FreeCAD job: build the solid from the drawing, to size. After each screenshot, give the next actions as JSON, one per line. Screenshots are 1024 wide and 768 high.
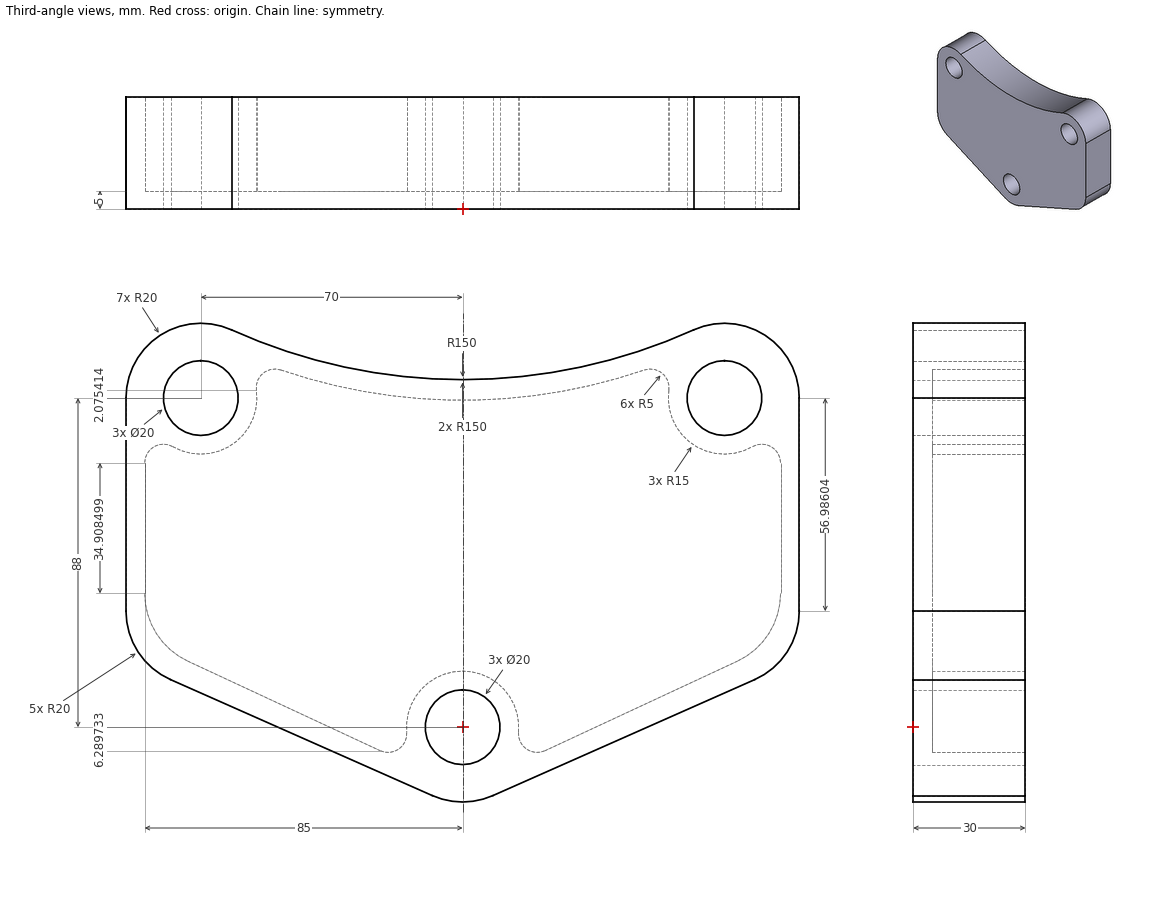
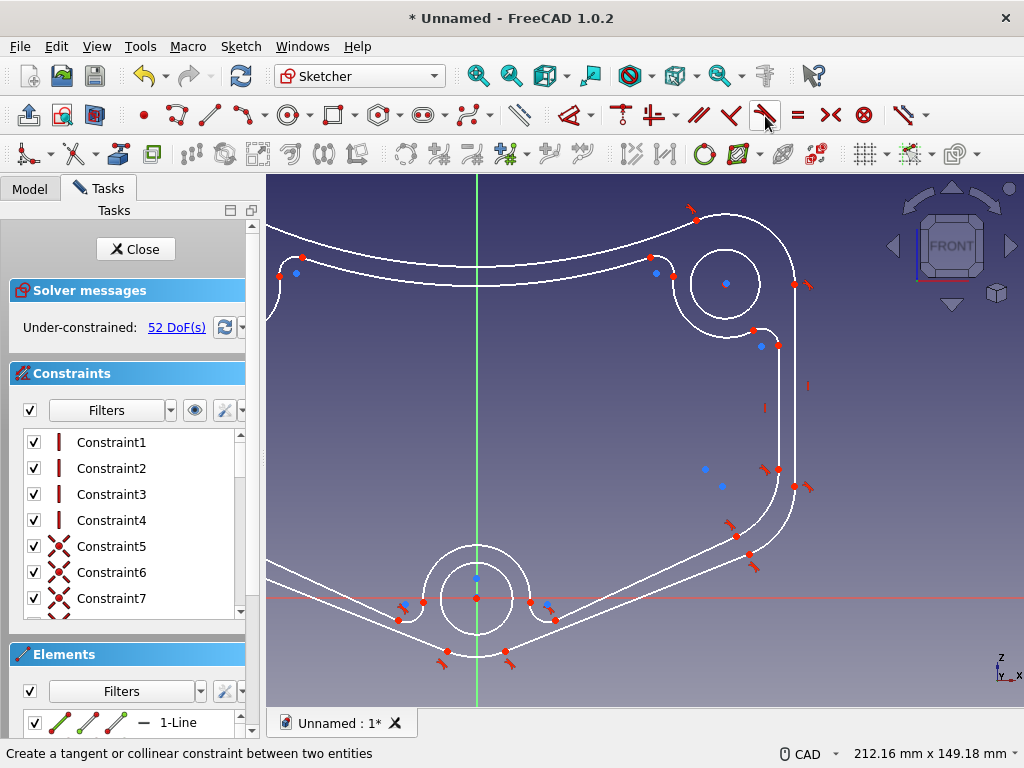
{"action": "left_click", "coordinate": [779, 433]}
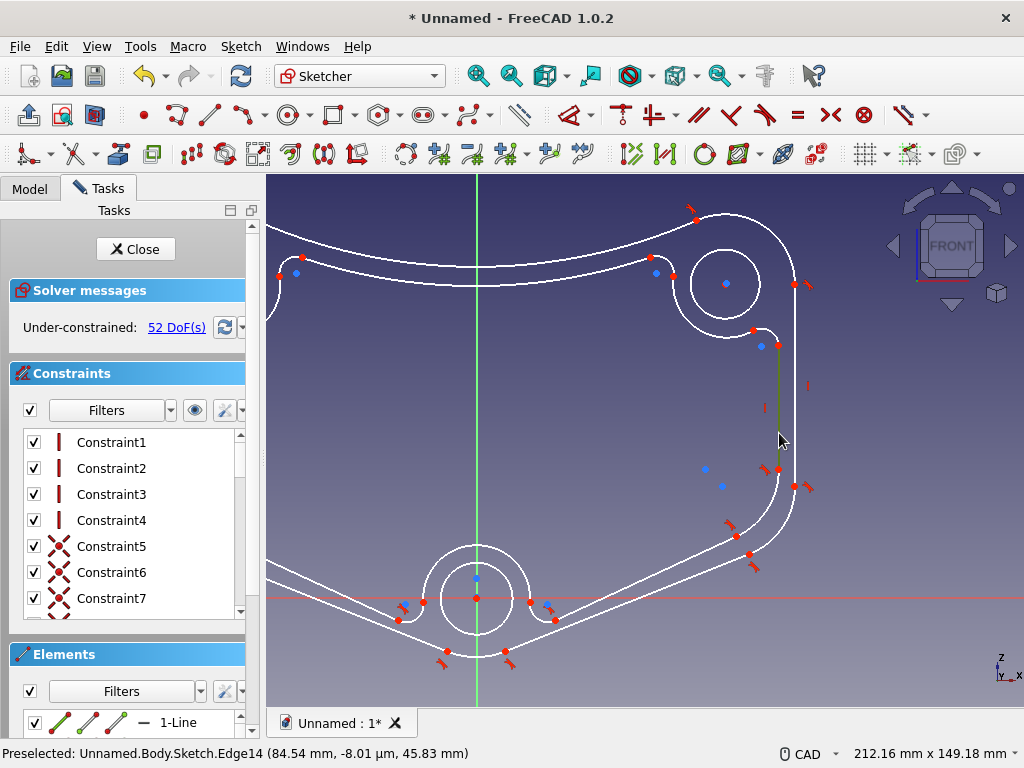
{"action": "scroll", "coordinate": [776, 336], "scroll_direction": "up", "scroll_amount": 2}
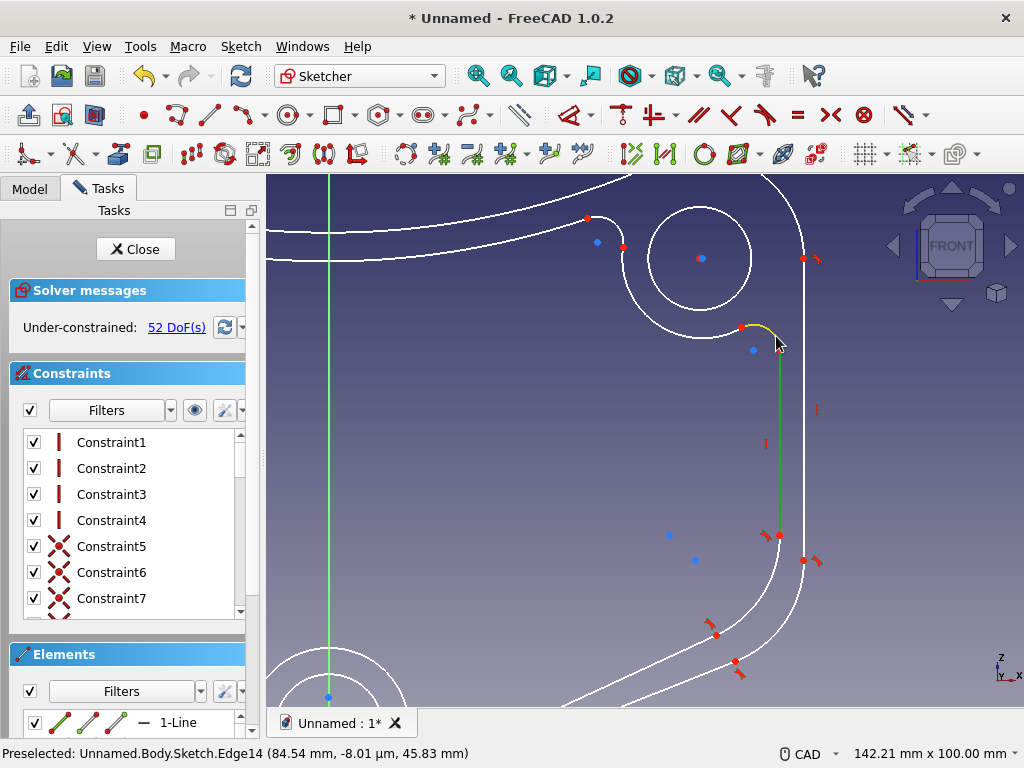
{"action": "left_click", "coordinate": [775, 336]}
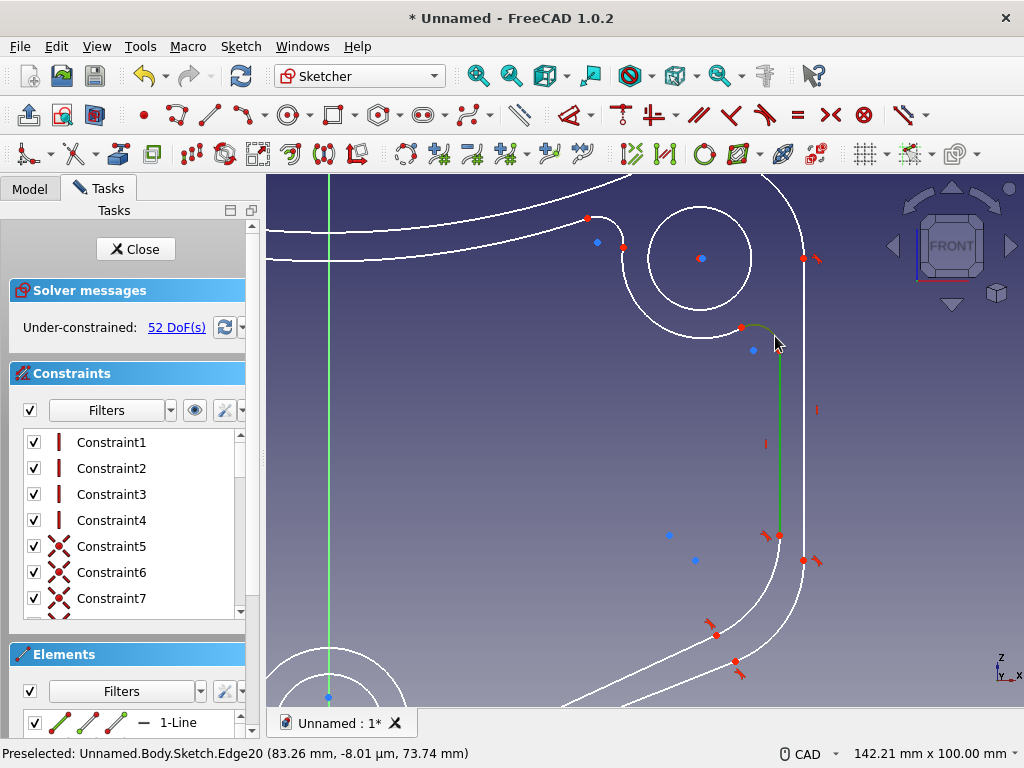
{"action": "left_click", "coordinate": [765, 116]}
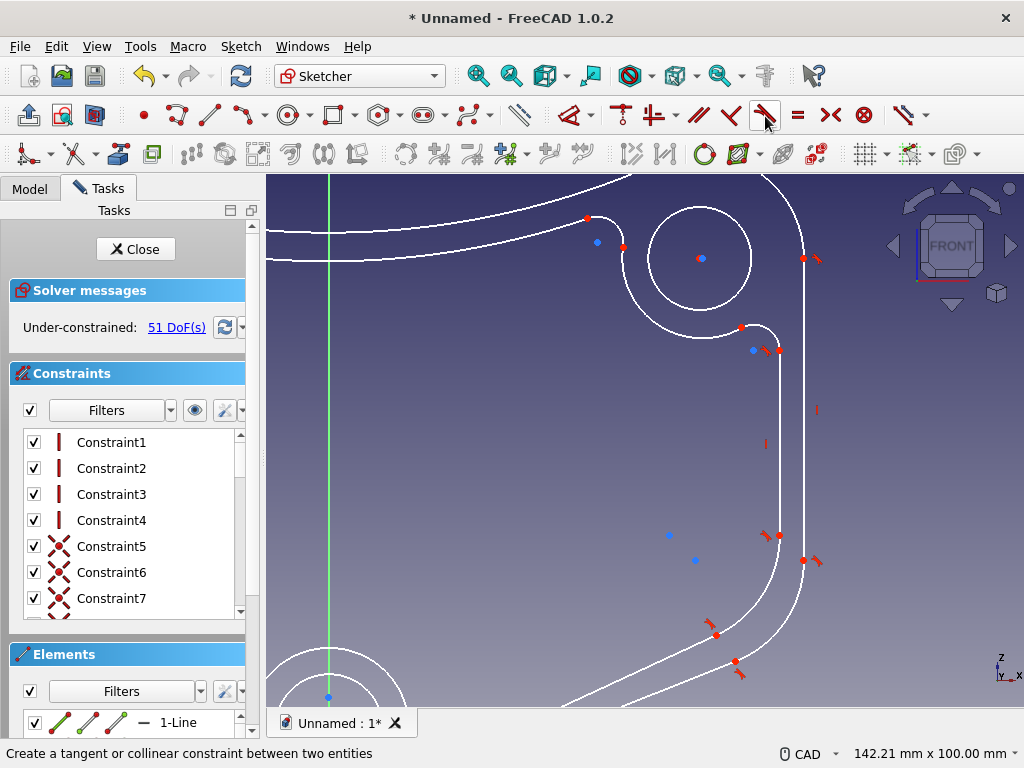
{"action": "scroll", "coordinate": [778, 395], "scroll_direction": "down", "scroll_amount": 4}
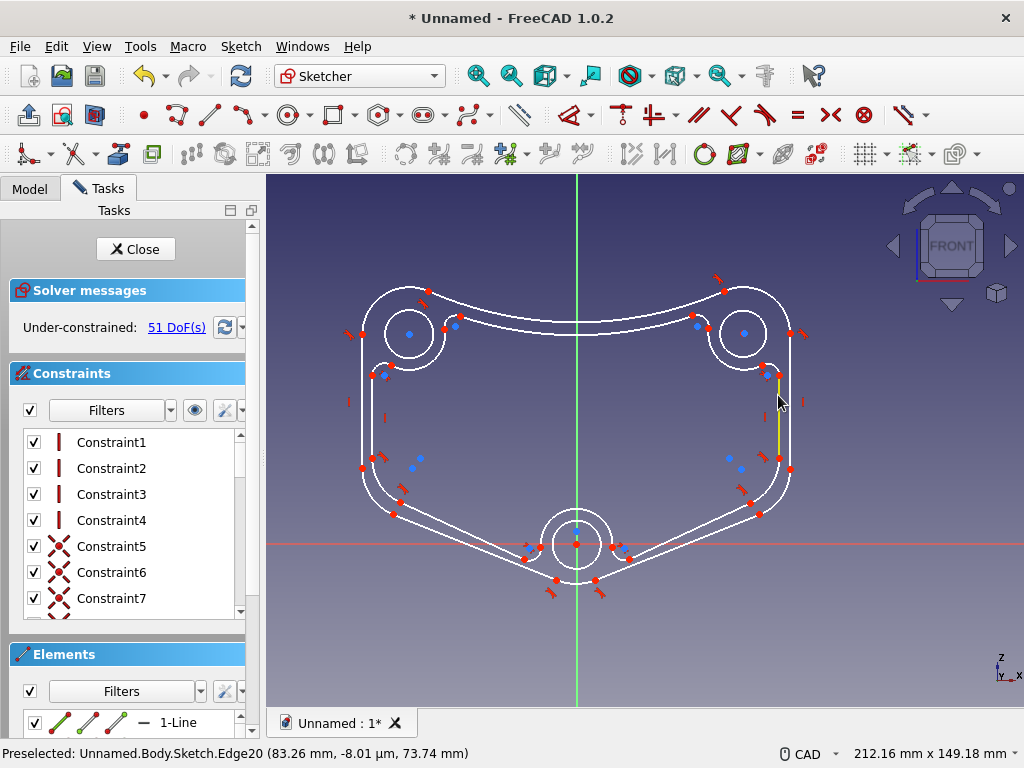
{"action": "scroll", "coordinate": [532, 560], "scroll_direction": "up", "scroll_amount": 4}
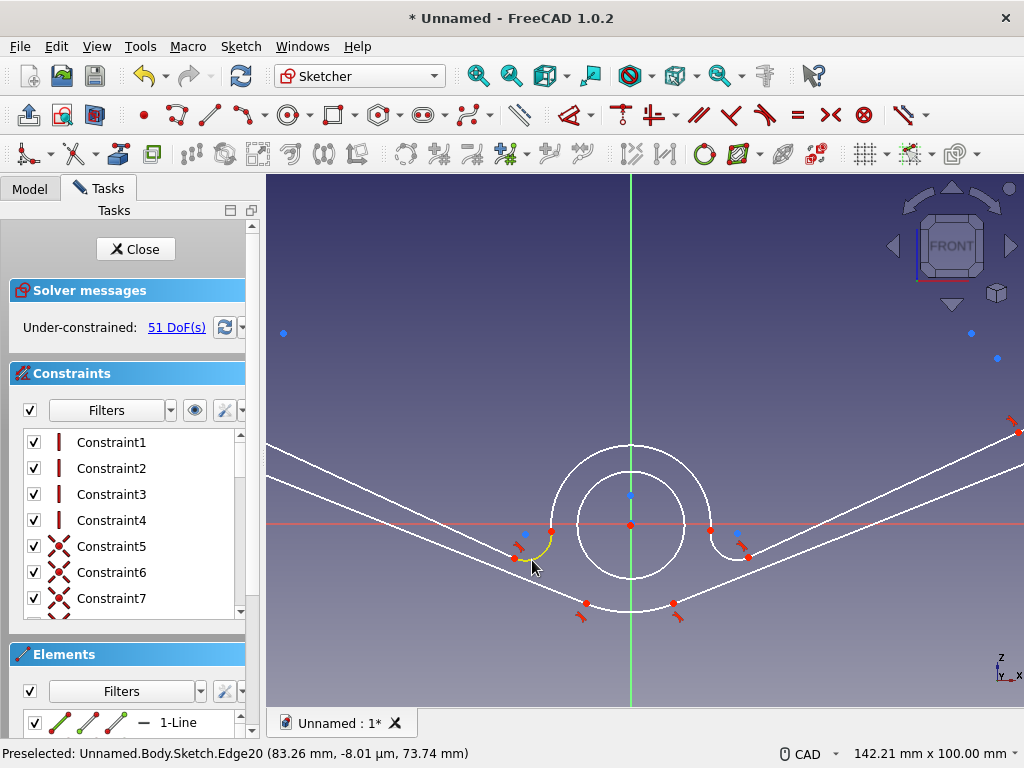
{"action": "left_click", "coordinate": [531, 560]}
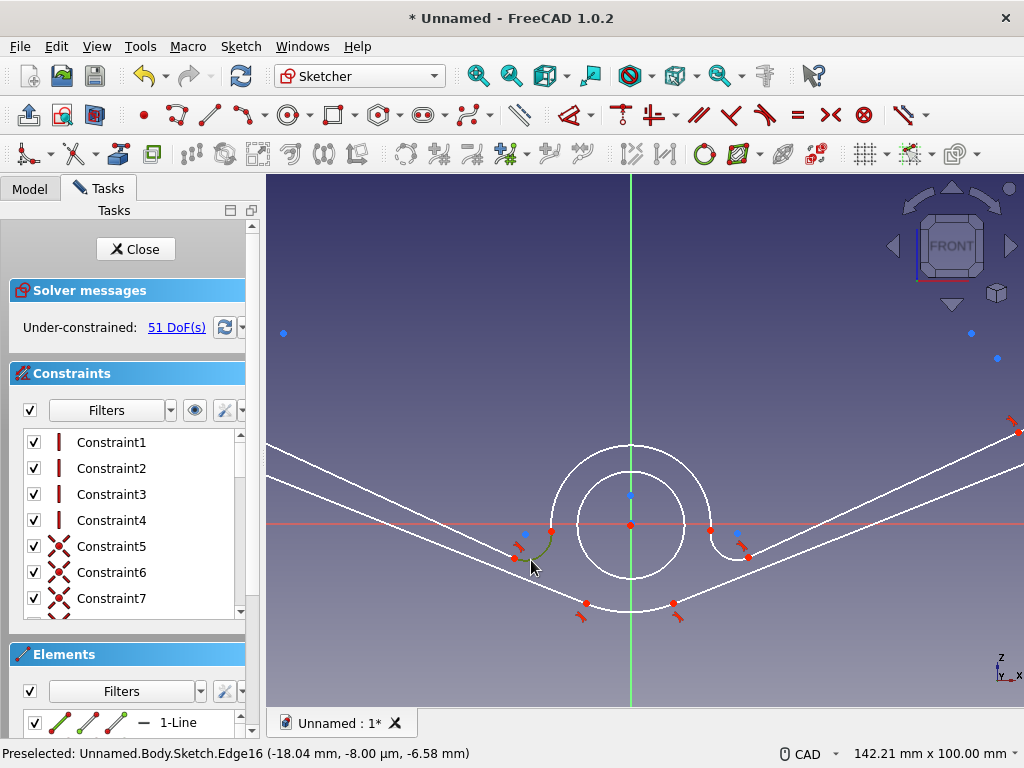
{"action": "left_click", "coordinate": [680, 462]}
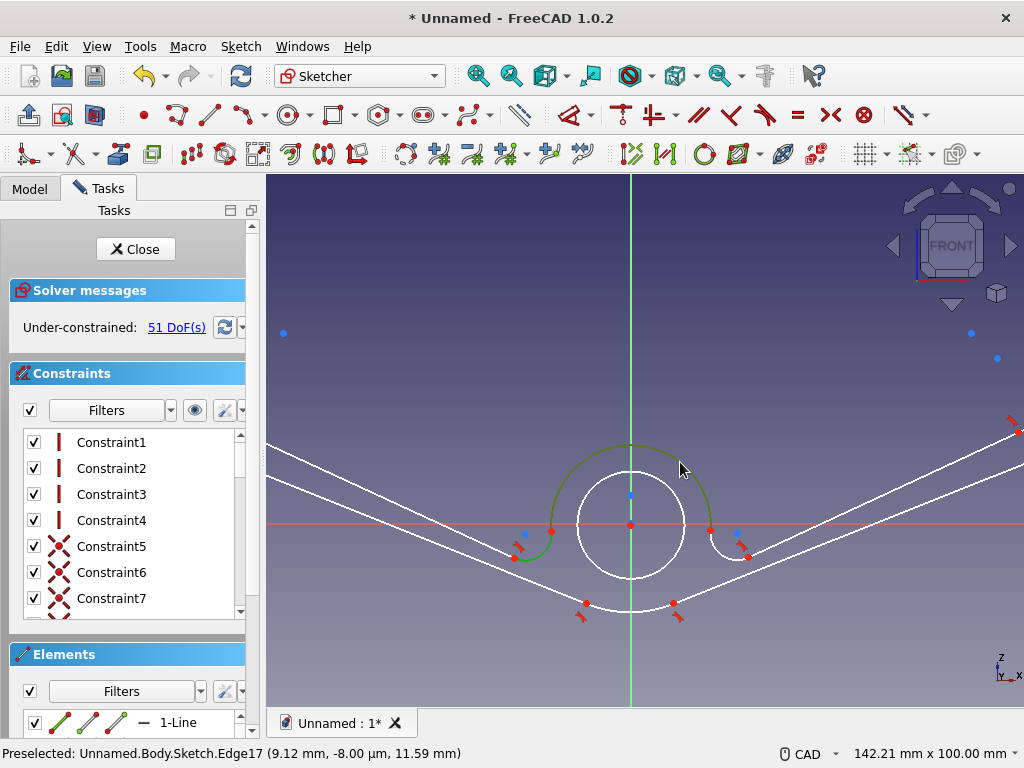
{"action": "left_click", "coordinate": [765, 116]}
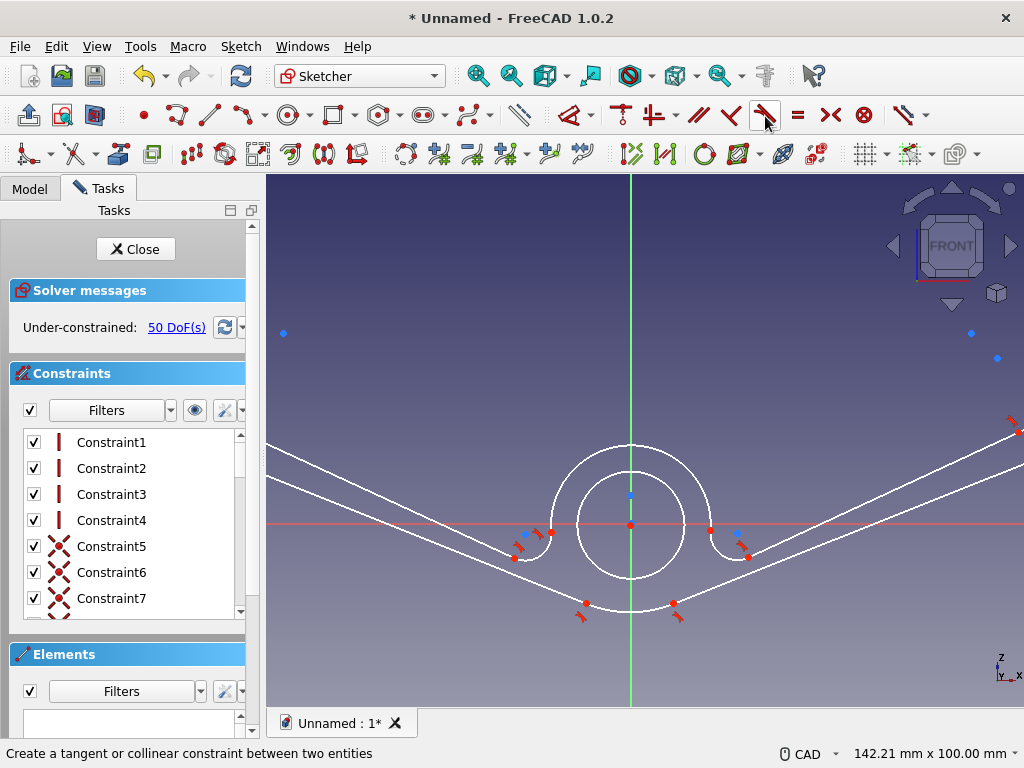
{"action": "left_click", "coordinate": [679, 462]}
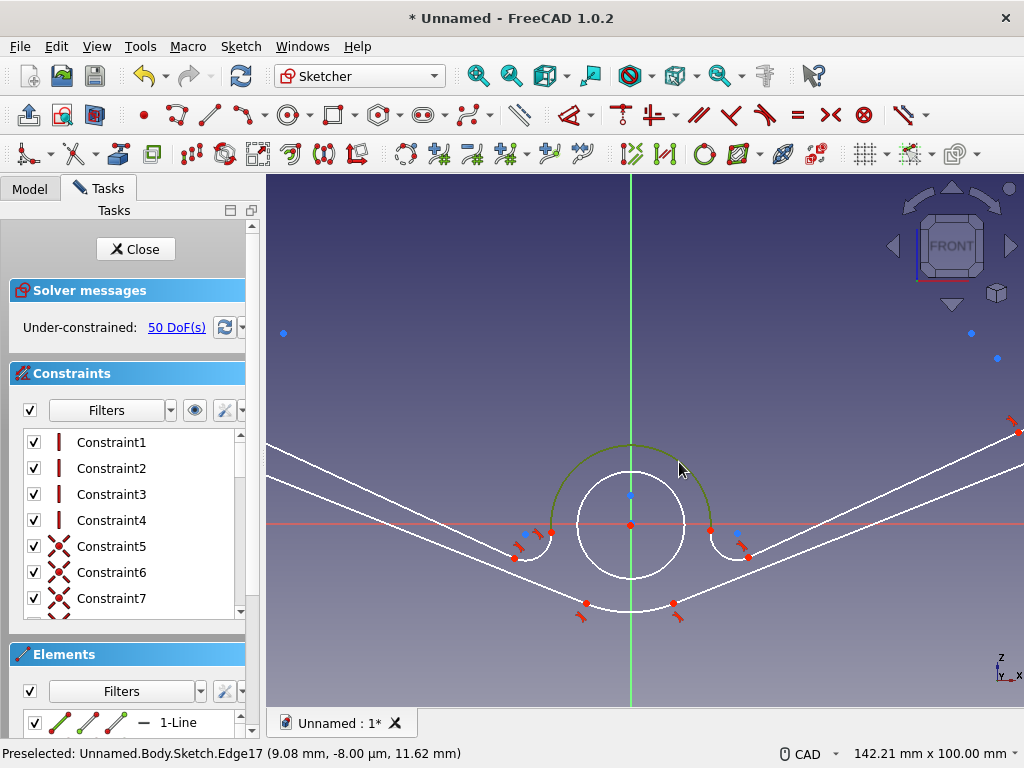
{"action": "left_click", "coordinate": [714, 547]}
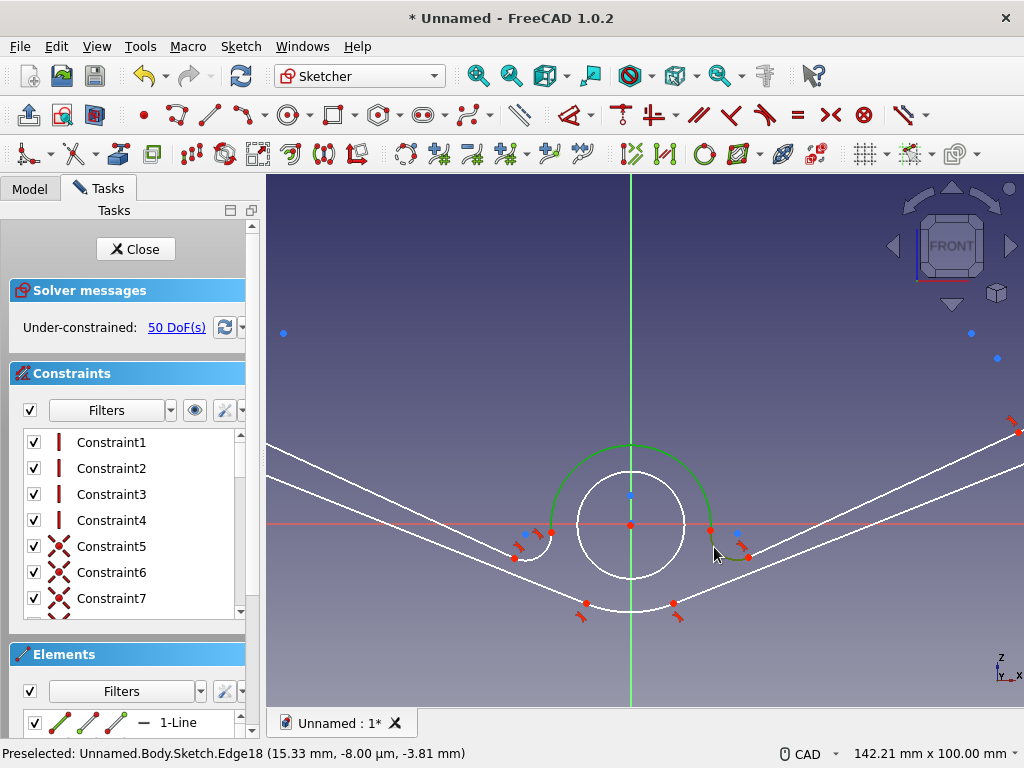
{"action": "key", "text": "t"}